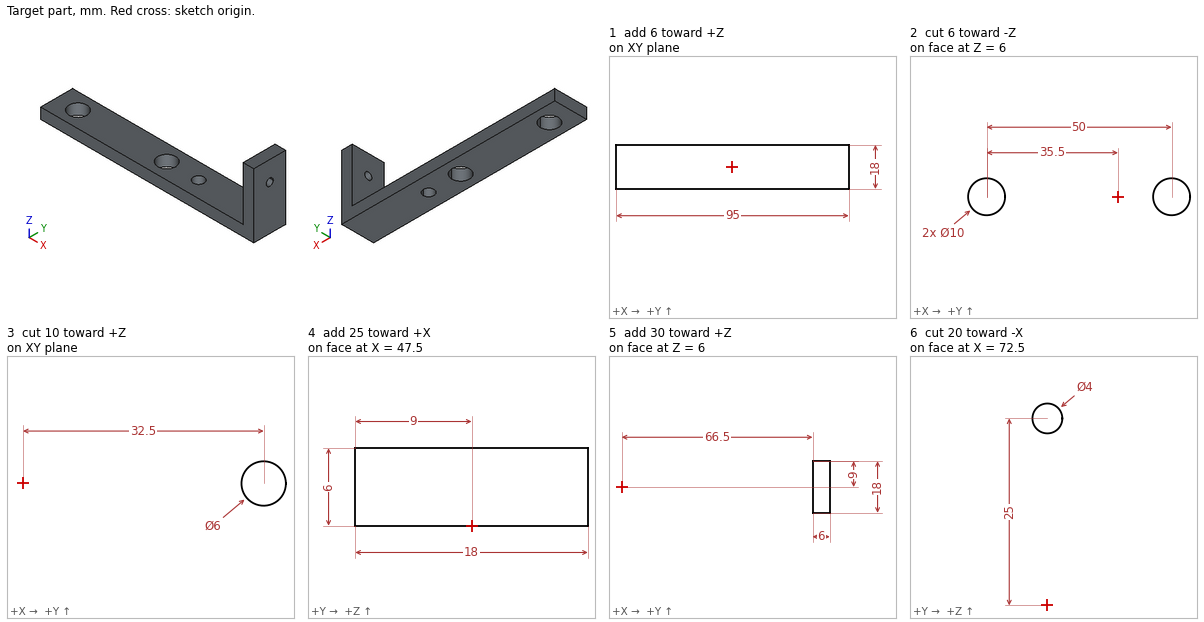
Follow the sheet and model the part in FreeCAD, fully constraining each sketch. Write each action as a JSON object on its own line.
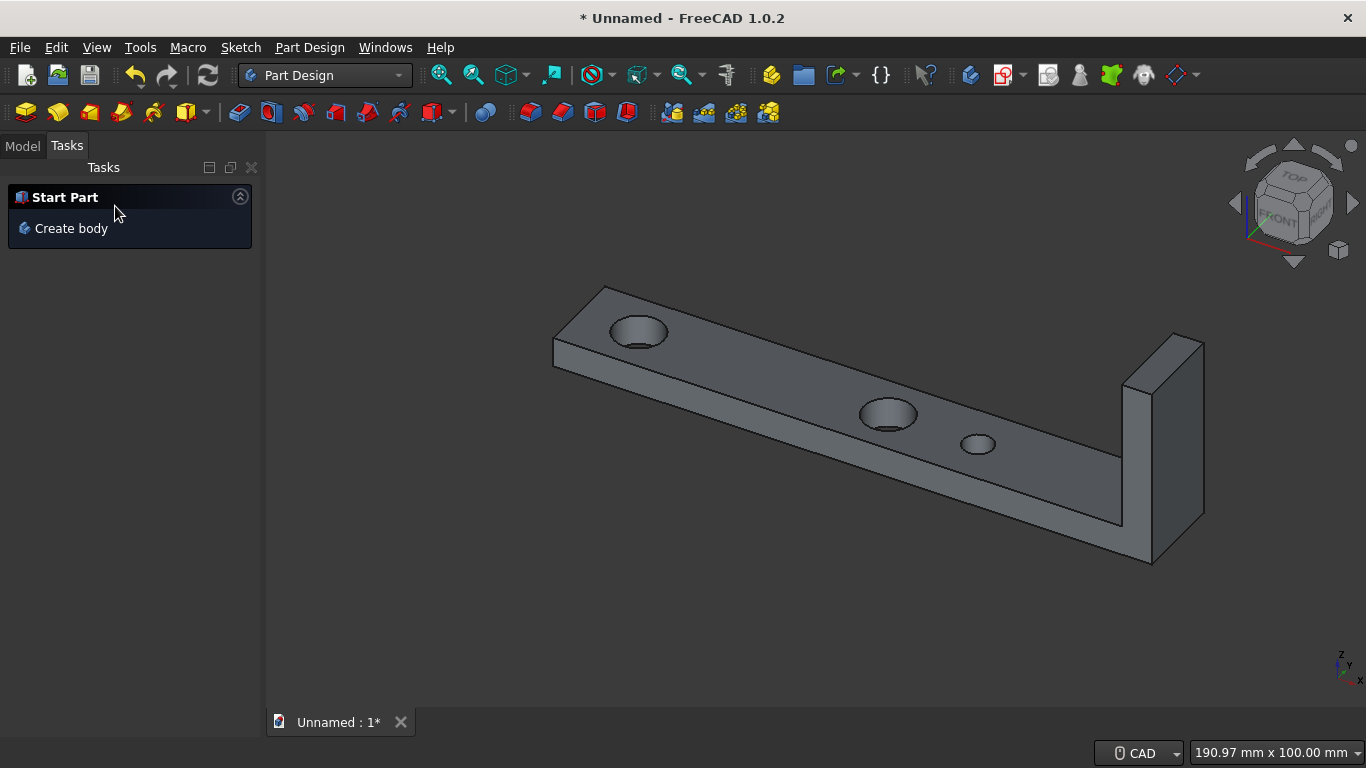
{"action": "left_click", "coordinate": [1178, 429]}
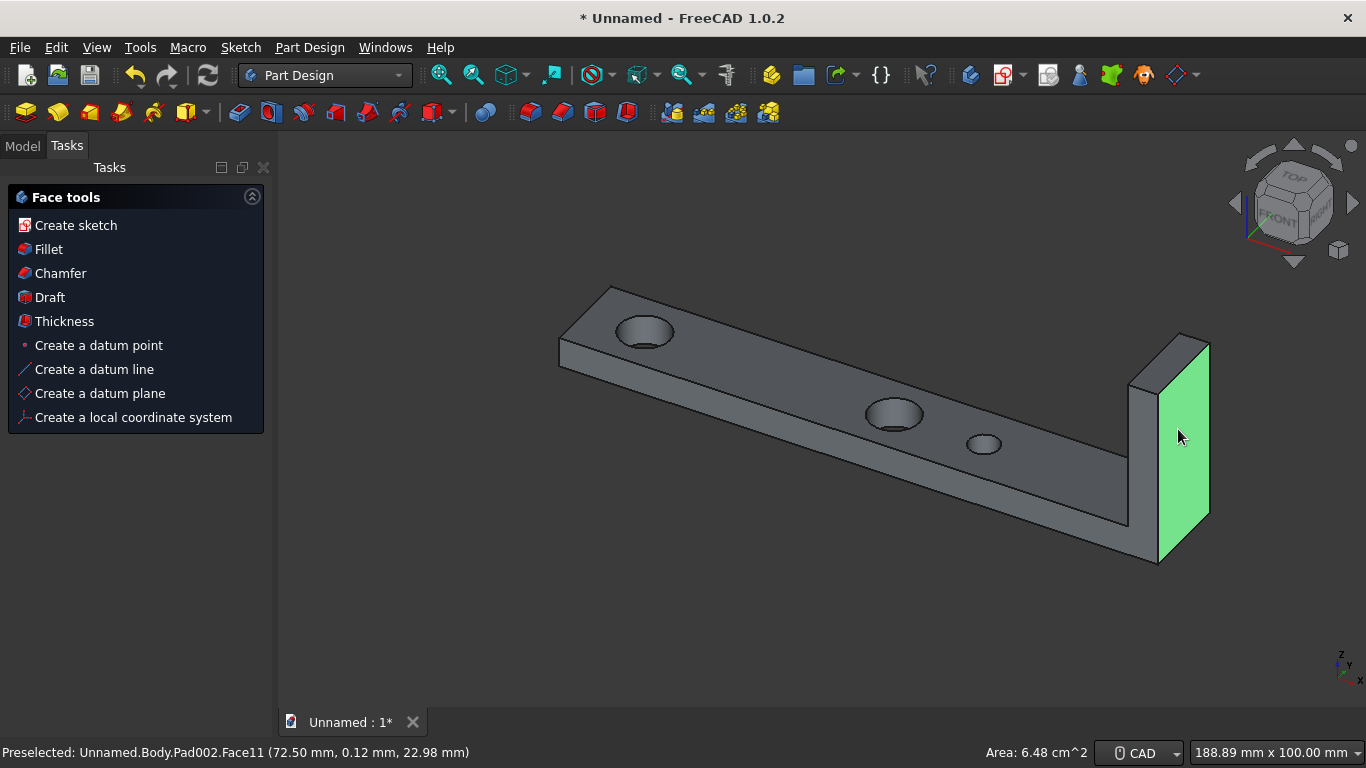
{"action": "left_click", "coordinate": [1004, 76]}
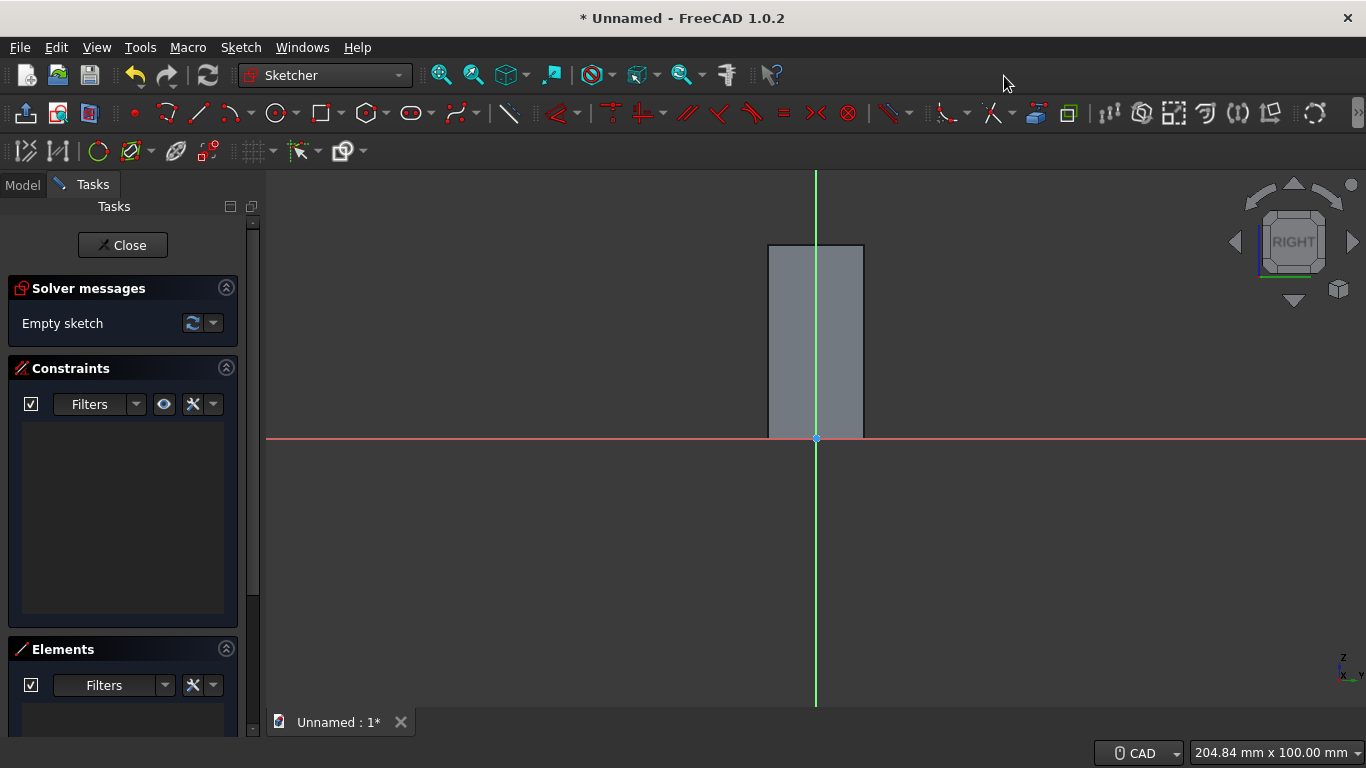
{"action": "scroll", "coordinate": [820, 296], "scroll_direction": "up", "scroll_amount": 14}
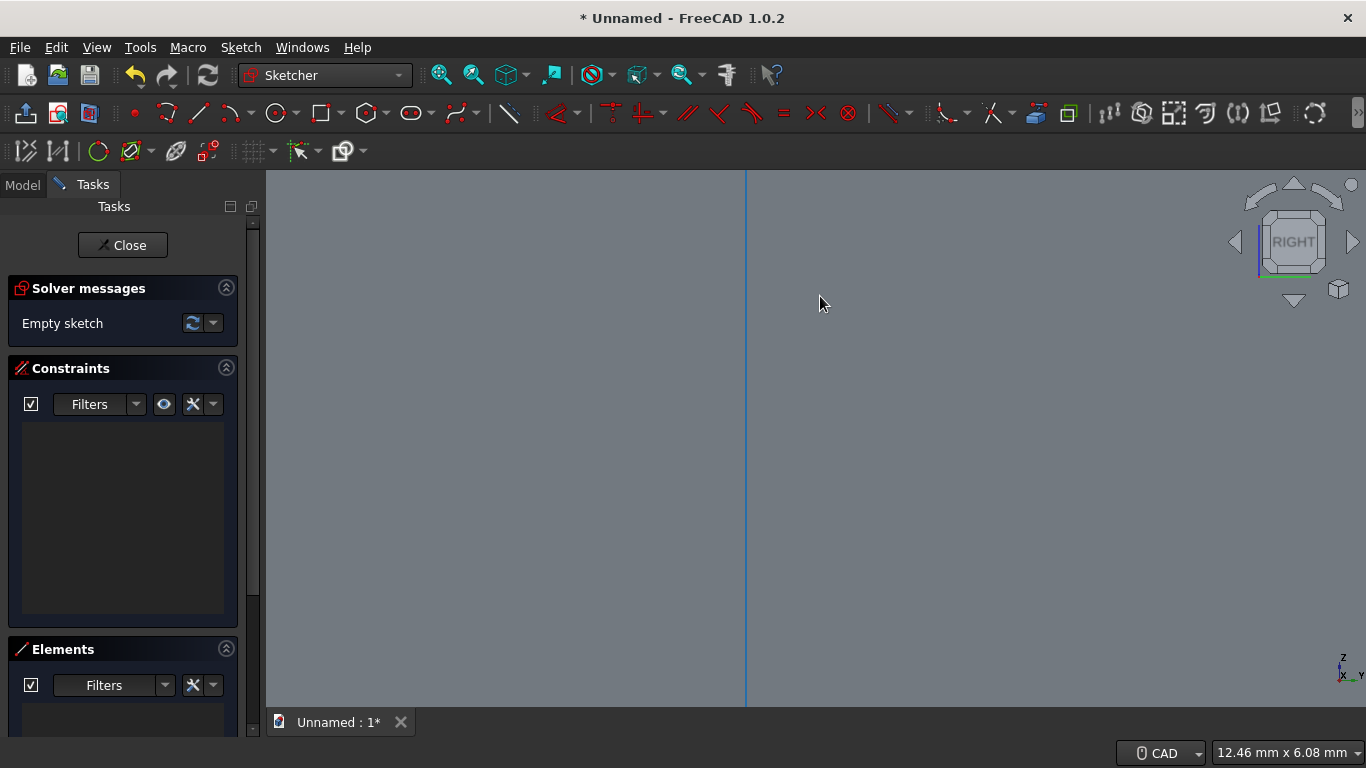
{"action": "left_click", "coordinate": [276, 114]}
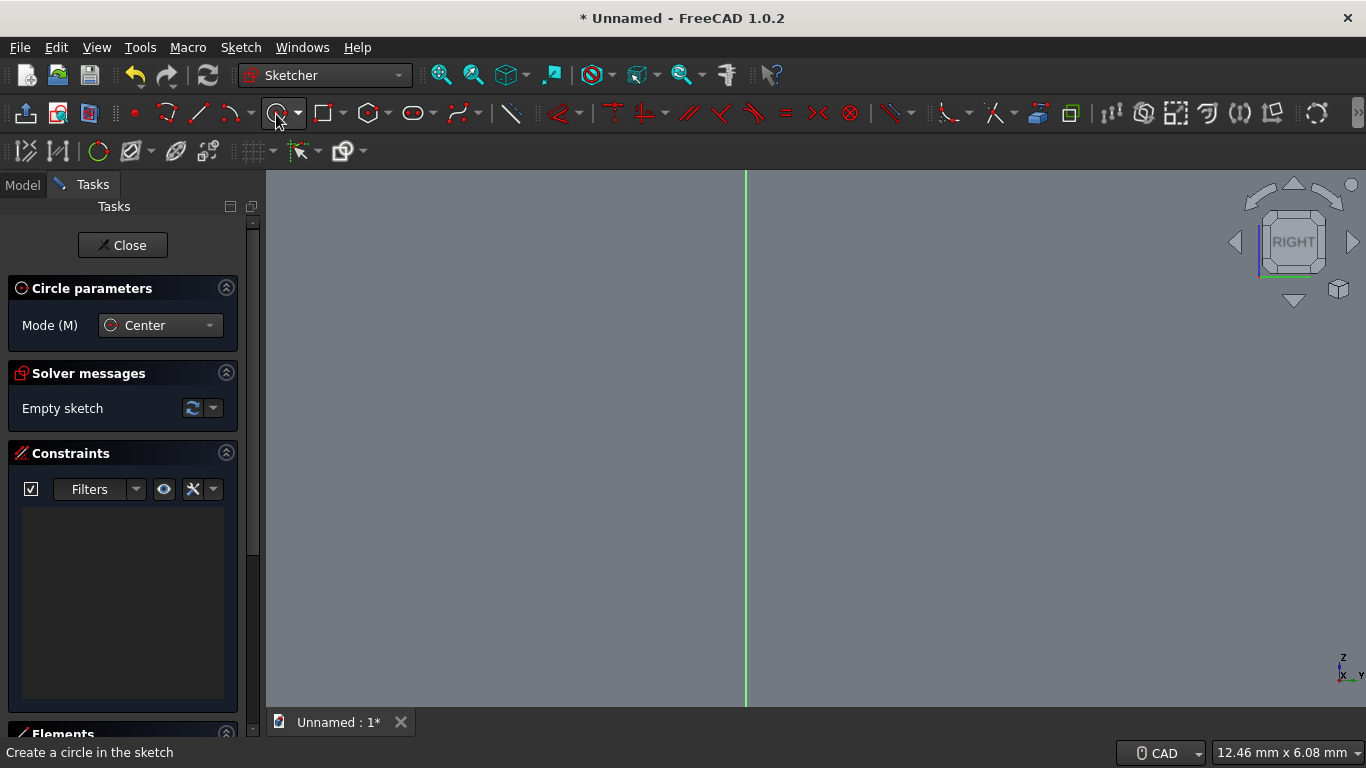
{"action": "left_click", "coordinate": [746, 428]}
{"action": "left_click", "coordinate": [871, 303]}
{"action": "key", "text": "Escape"}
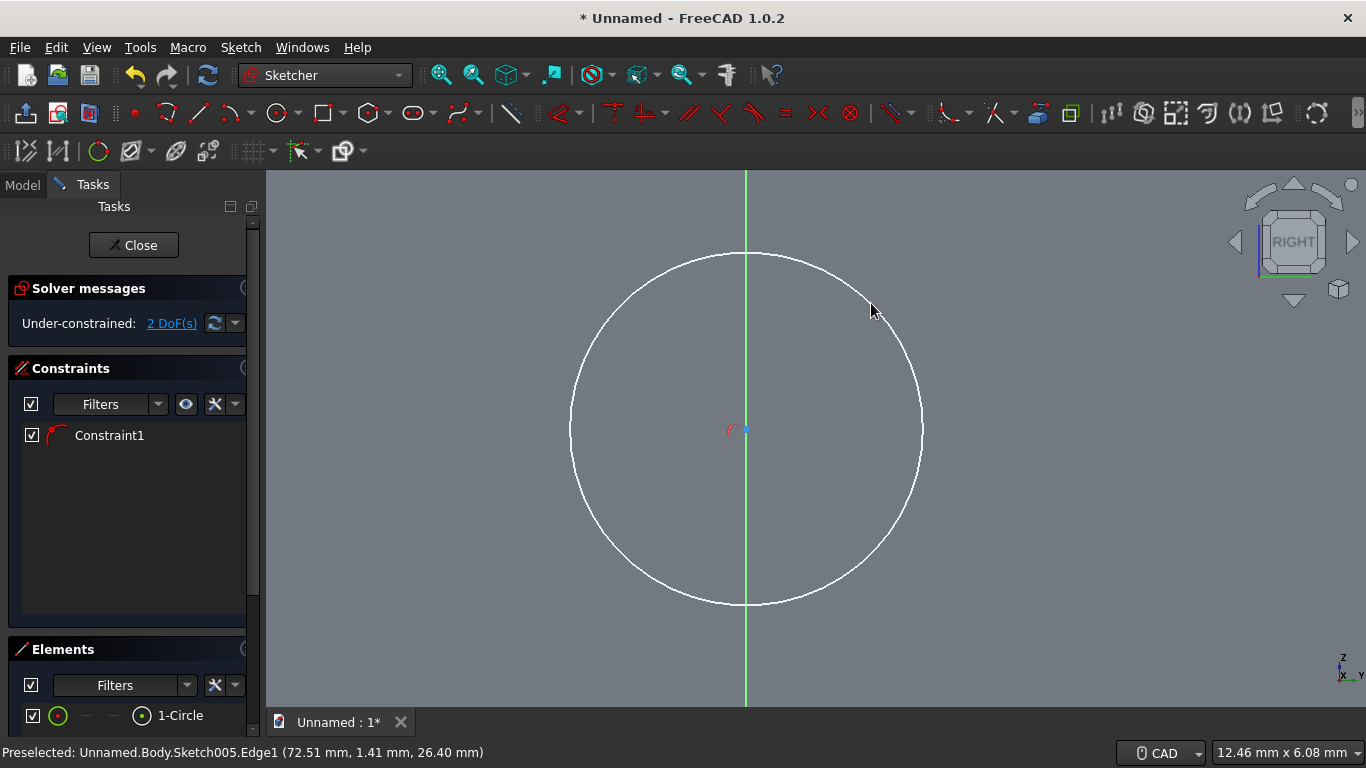
{"action": "left_click", "coordinate": [558, 114]}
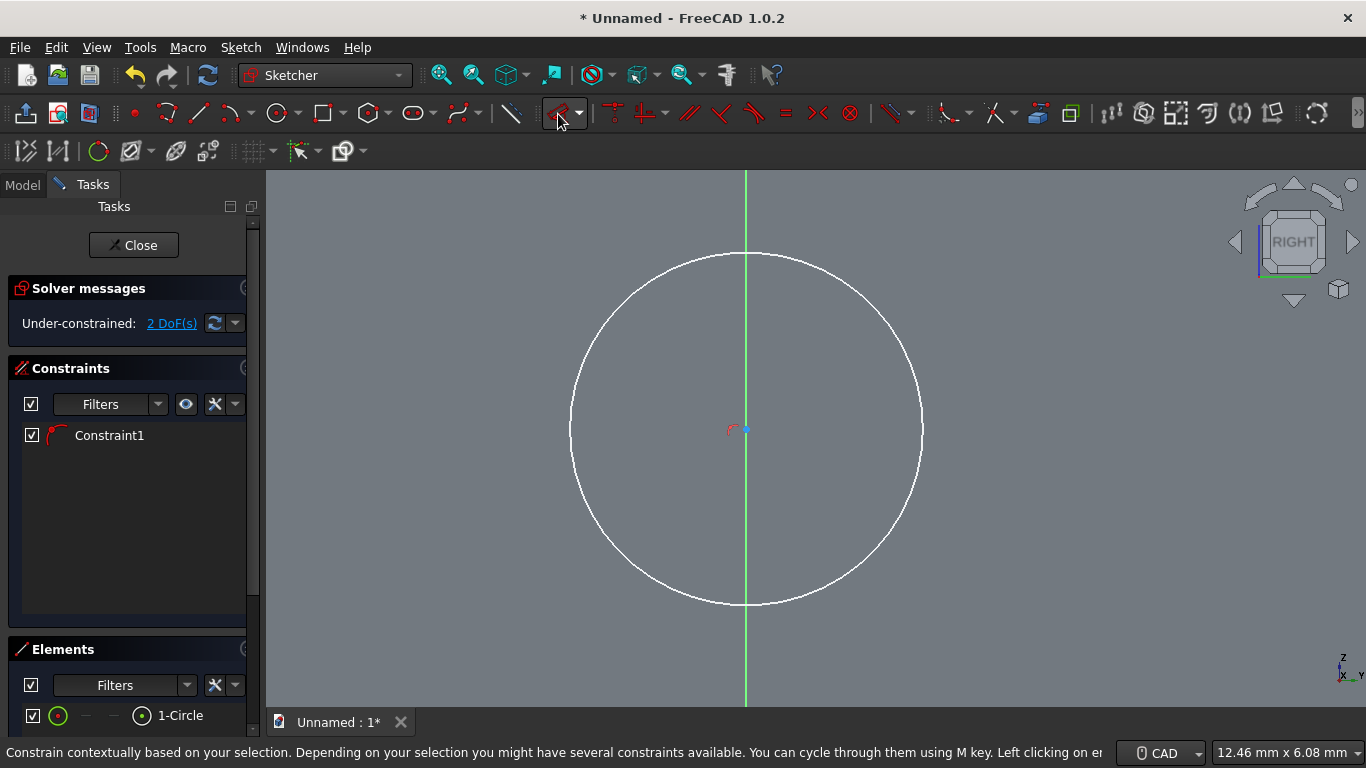
{"action": "left_click", "coordinate": [871, 304]}
{"action": "left_click", "coordinate": [894, 281]}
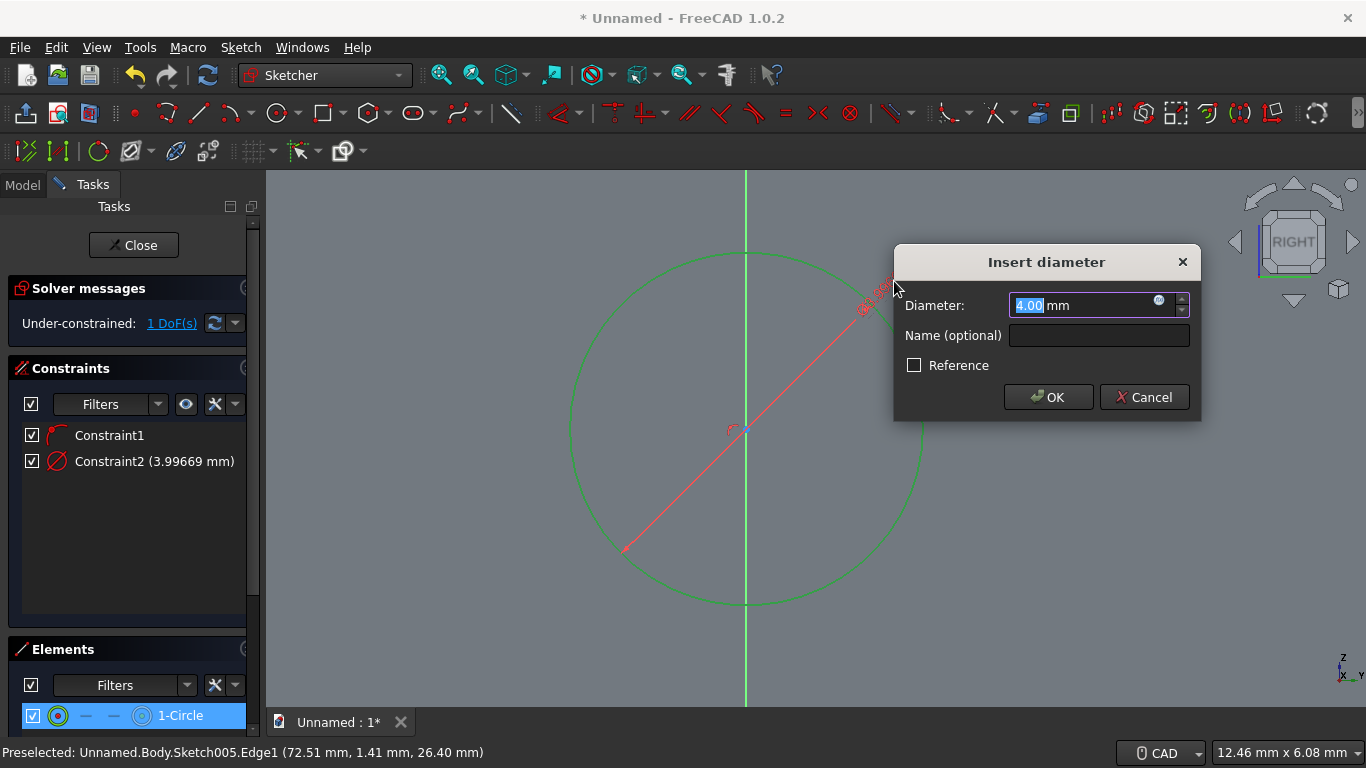
{"action": "type", "text": "4"}
{"action": "key", "text": "Return"}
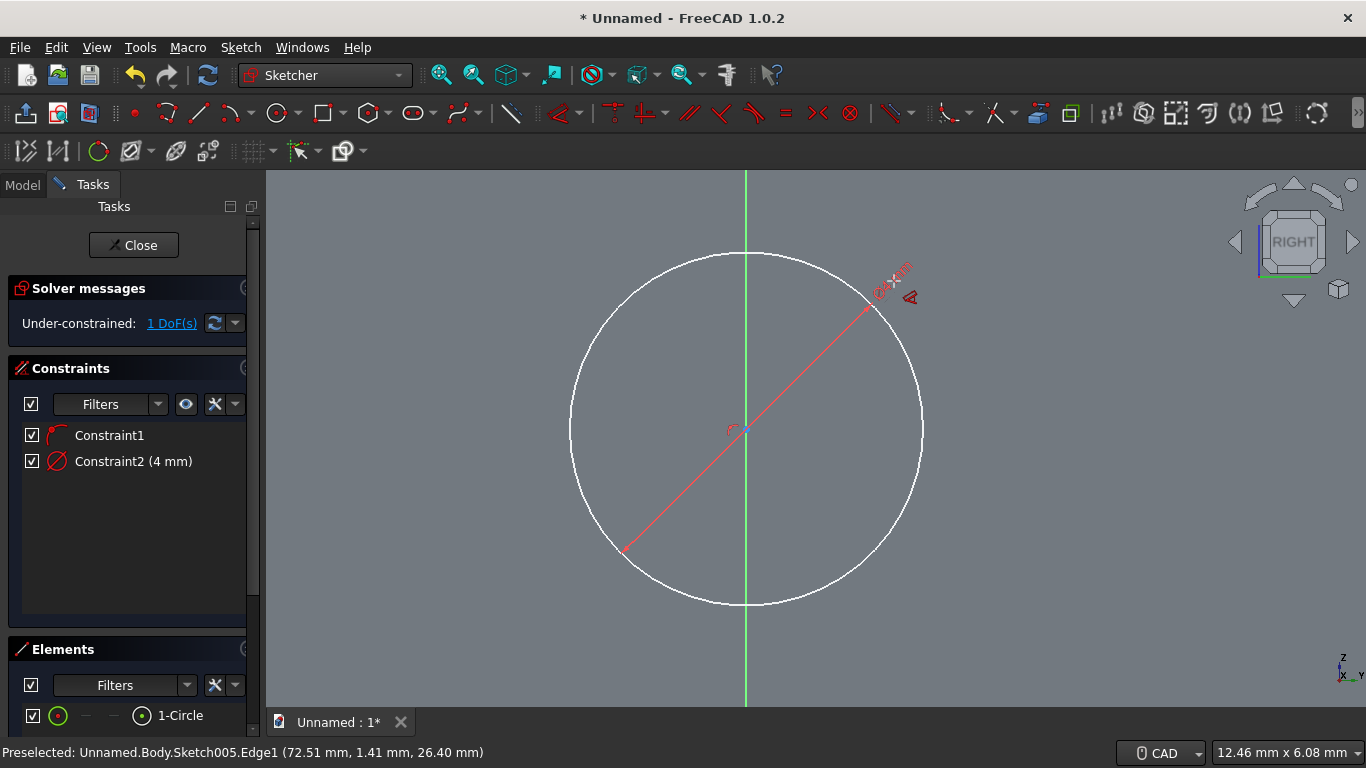
{"action": "left_click", "coordinate": [746, 429]}
{"action": "left_click", "coordinate": [780, 554]}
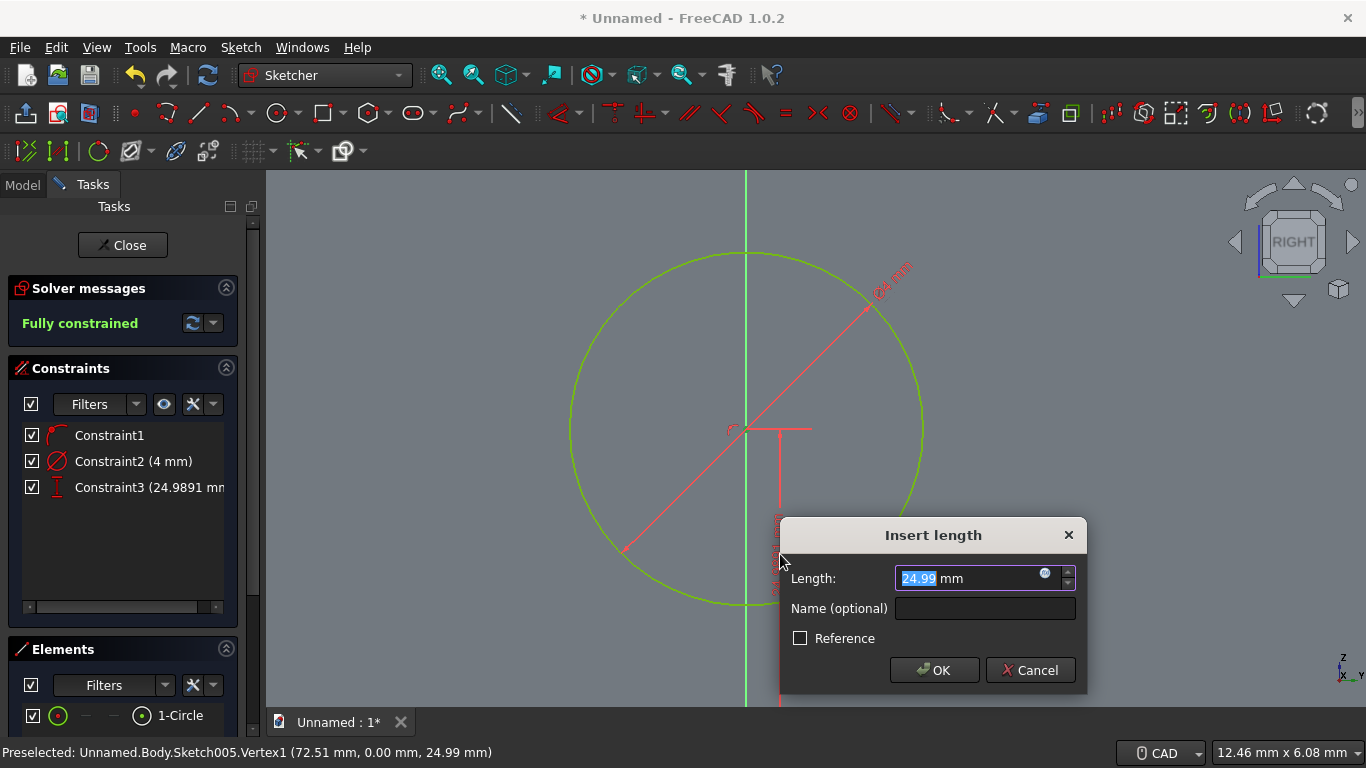
{"action": "type", "text": "25"}
{"action": "key", "text": "Return"}
{"action": "key", "text": "Escape"}